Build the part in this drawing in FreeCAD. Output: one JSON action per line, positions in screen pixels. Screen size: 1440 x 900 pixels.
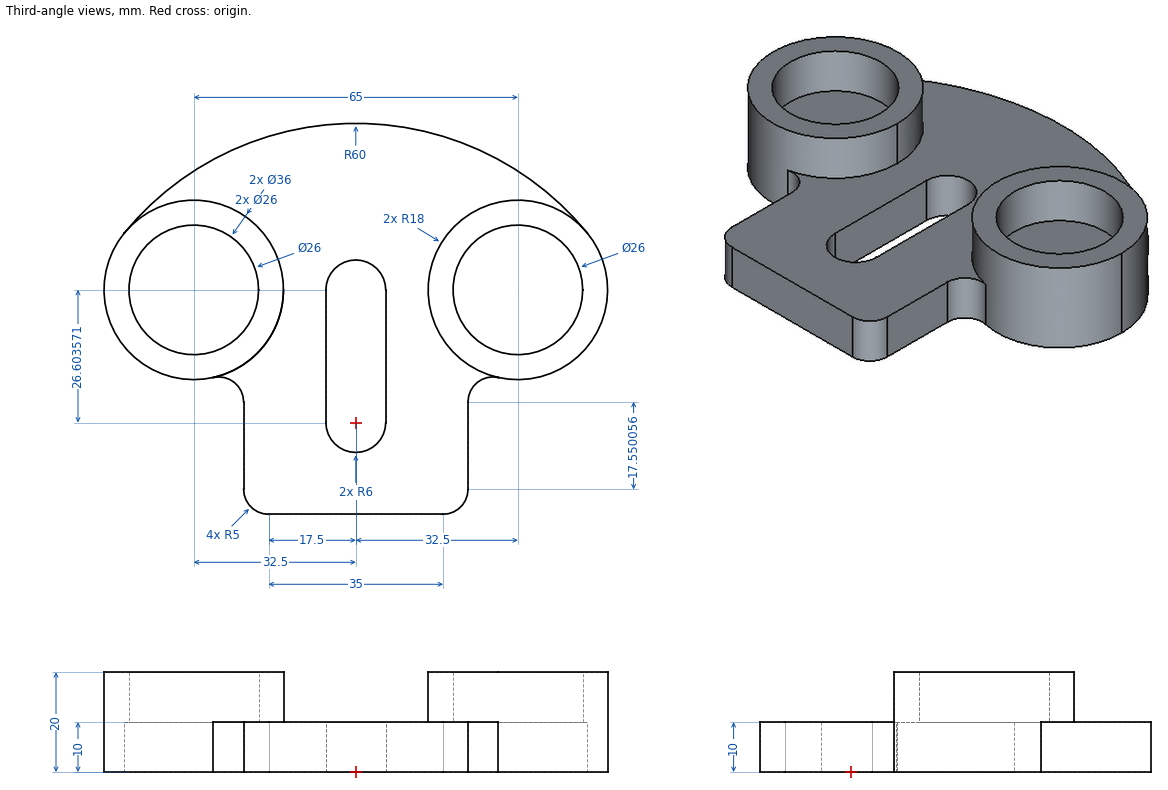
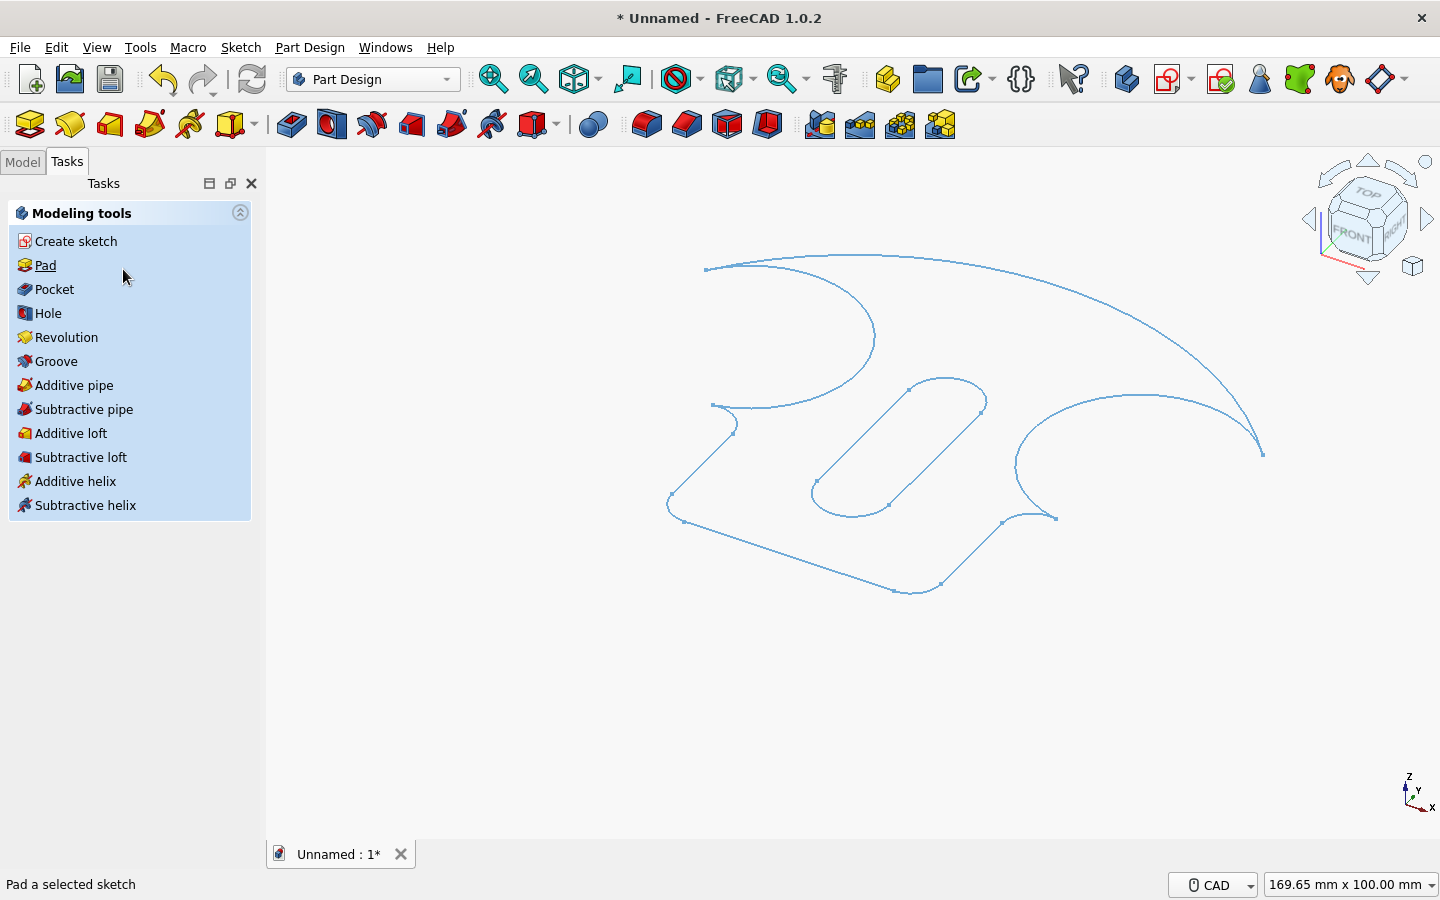
{"action": "left_click", "coordinate": [30, 124]}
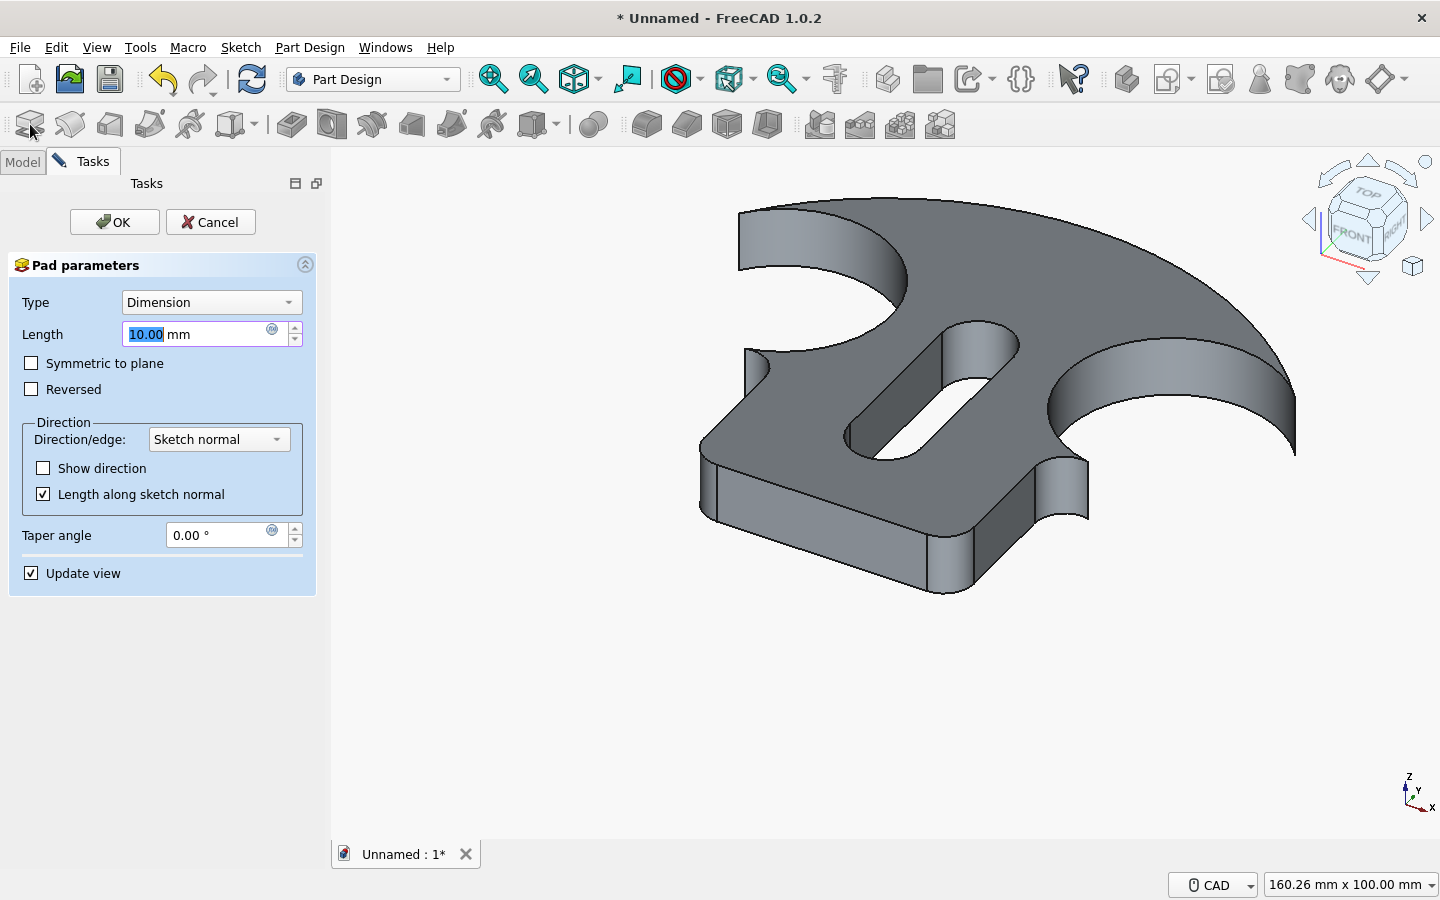
{"action": "type", "text": "10"}
{"action": "key", "text": "Tab"}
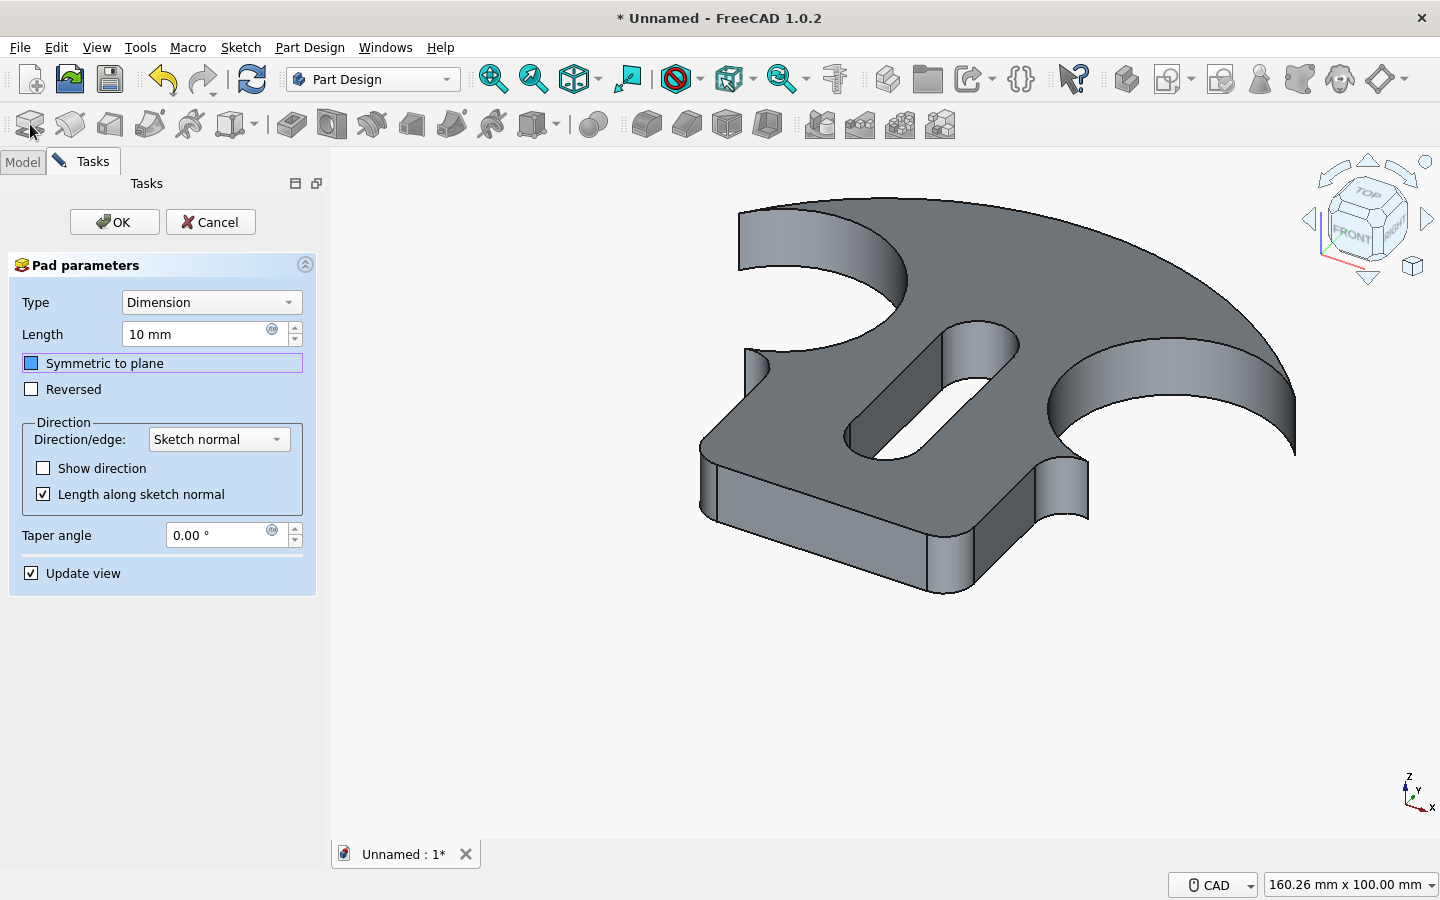
{"action": "left_click", "coordinate": [115, 222]}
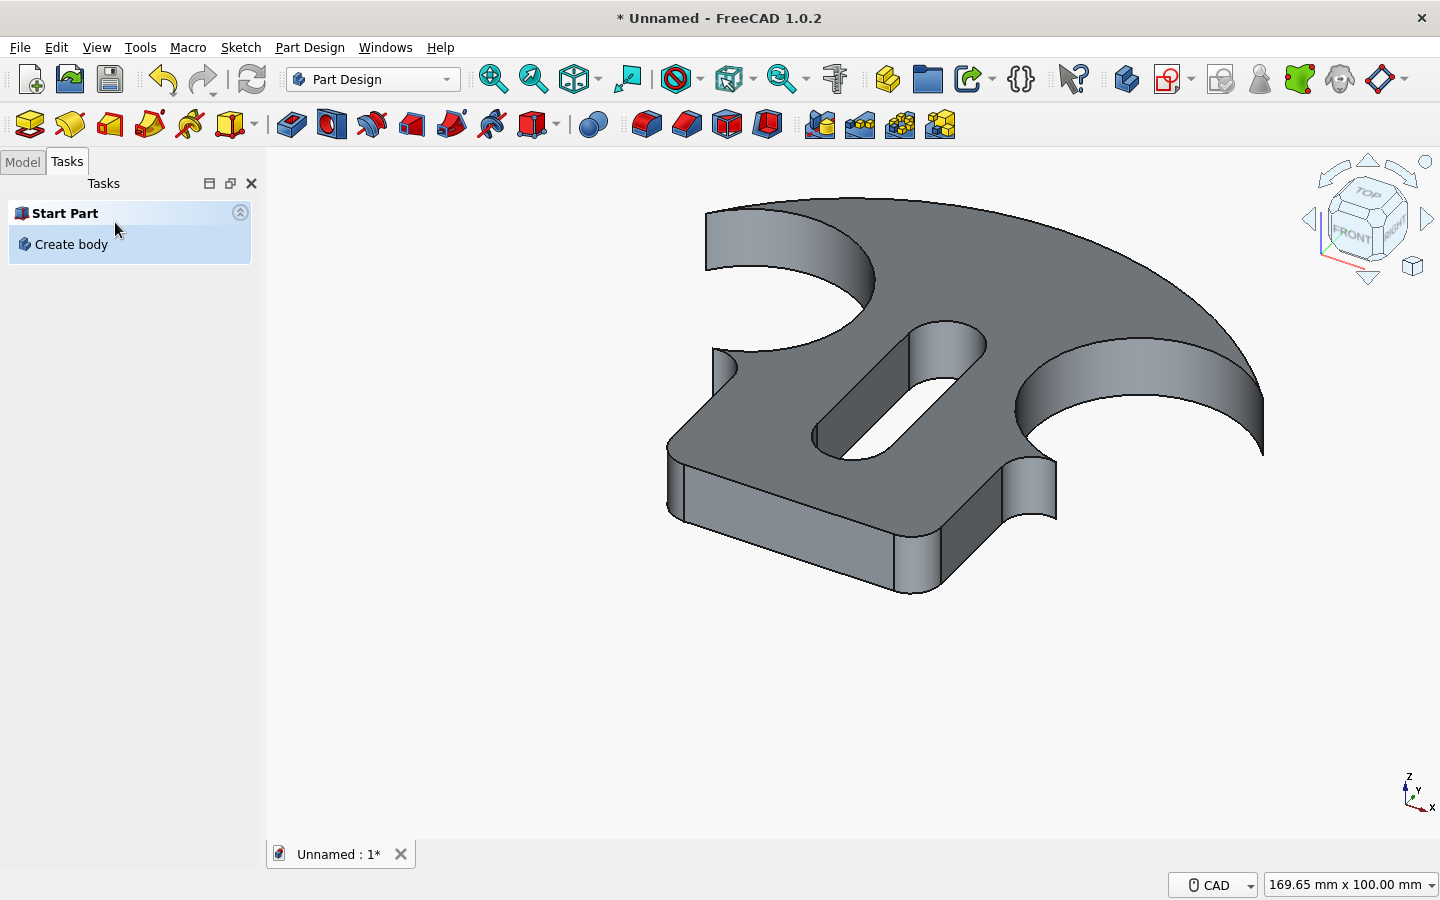
{"action": "left_click", "coordinate": [494, 80]}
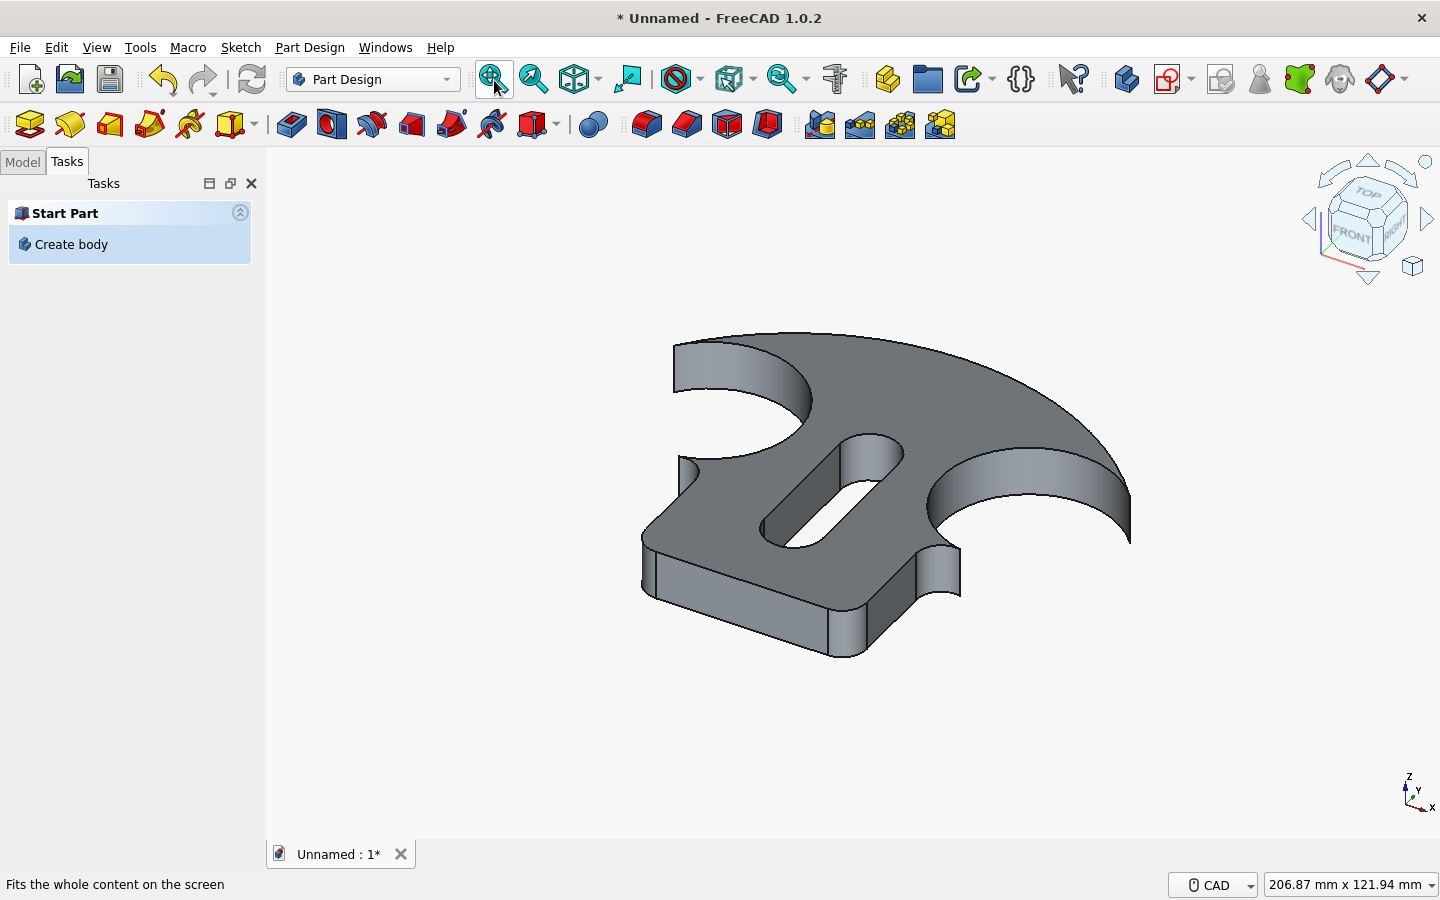
{"action": "left_click", "coordinate": [1128, 80]}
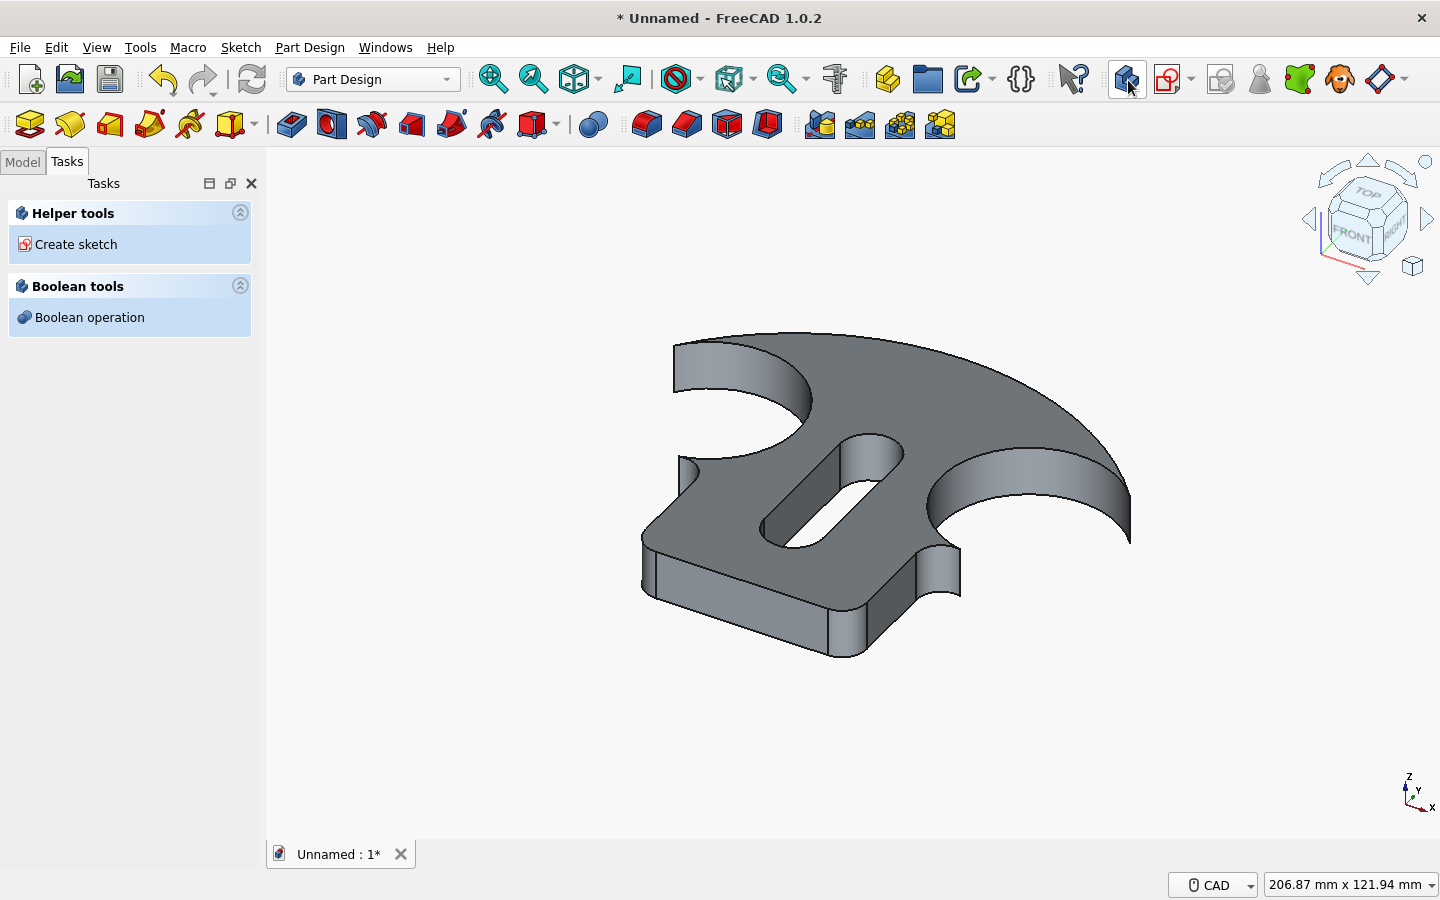
{"action": "left_click", "coordinate": [306, 799]}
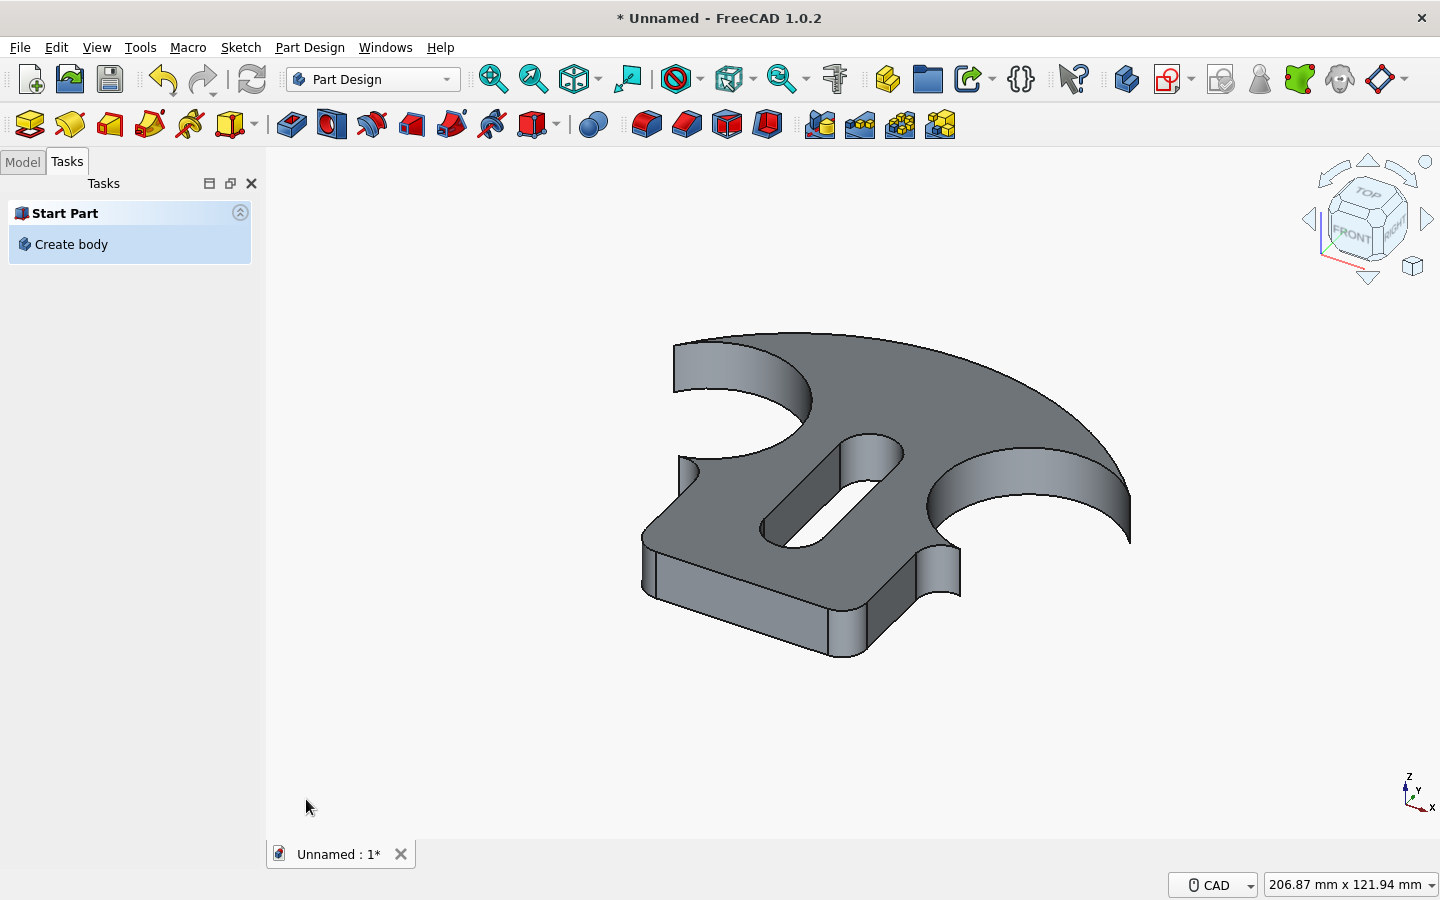
{"action": "left_click", "coordinate": [1168, 80]}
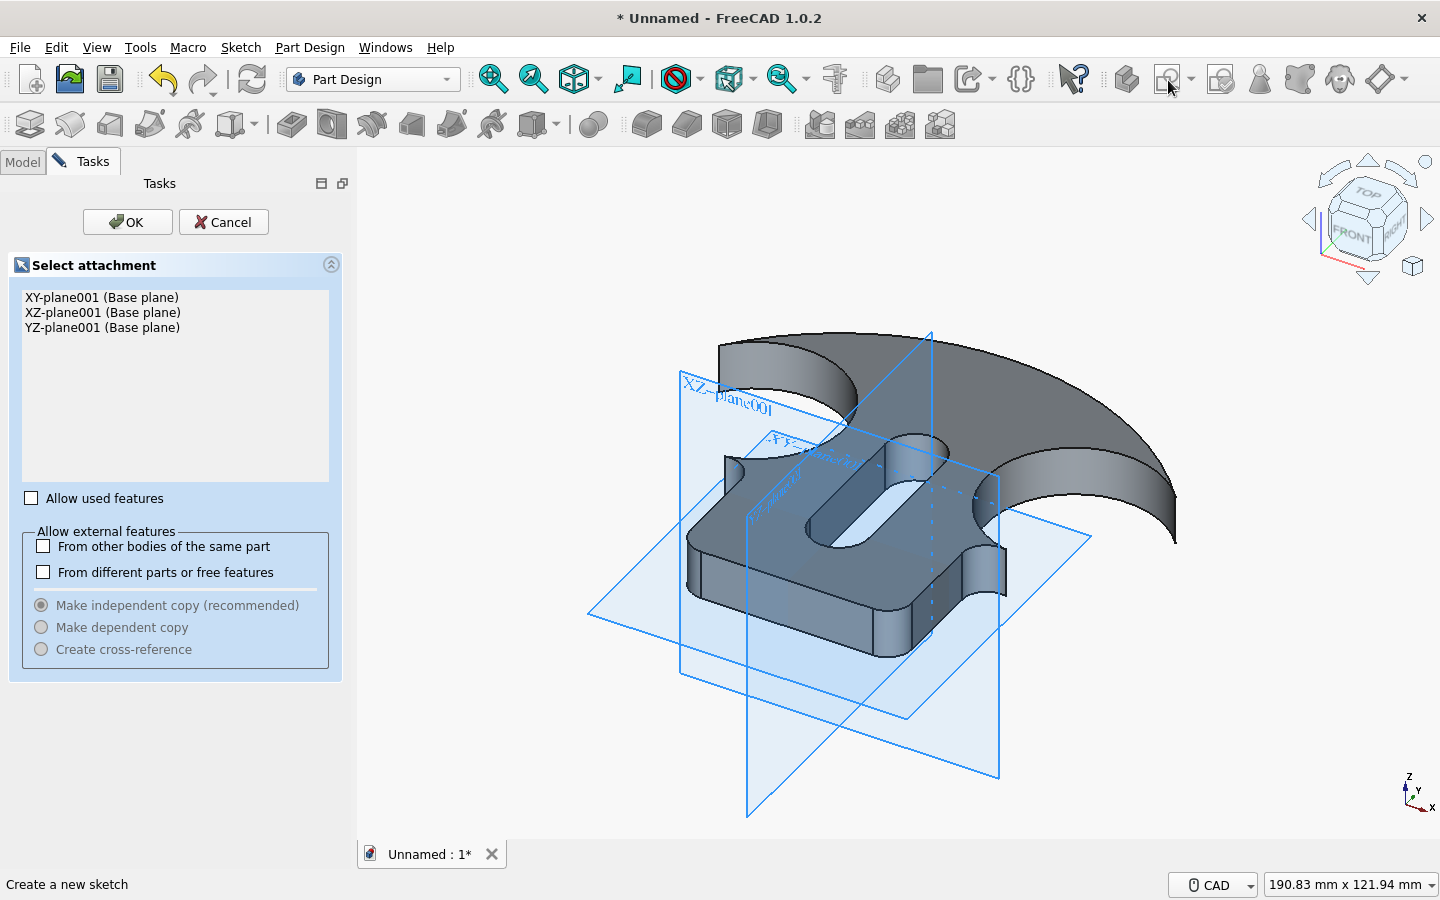
{"action": "left_click", "coordinate": [82, 298]}